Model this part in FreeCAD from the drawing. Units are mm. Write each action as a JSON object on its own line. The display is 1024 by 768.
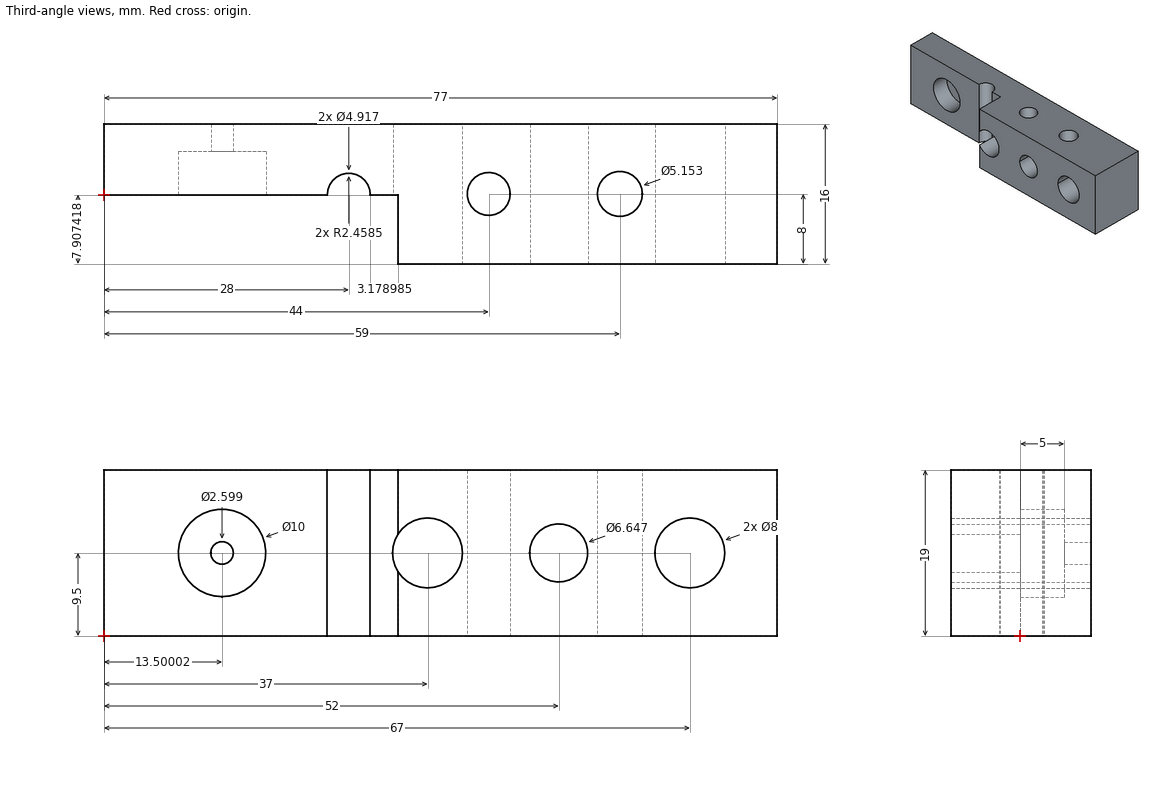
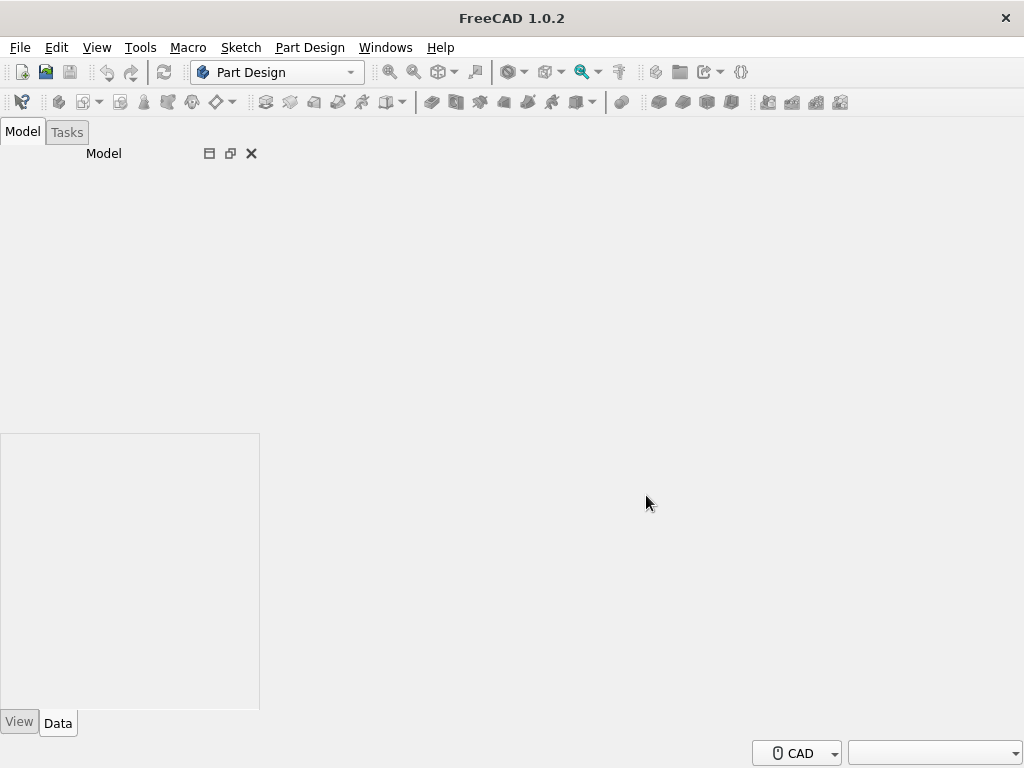
{"action": "left_click", "coordinate": [22, 72]}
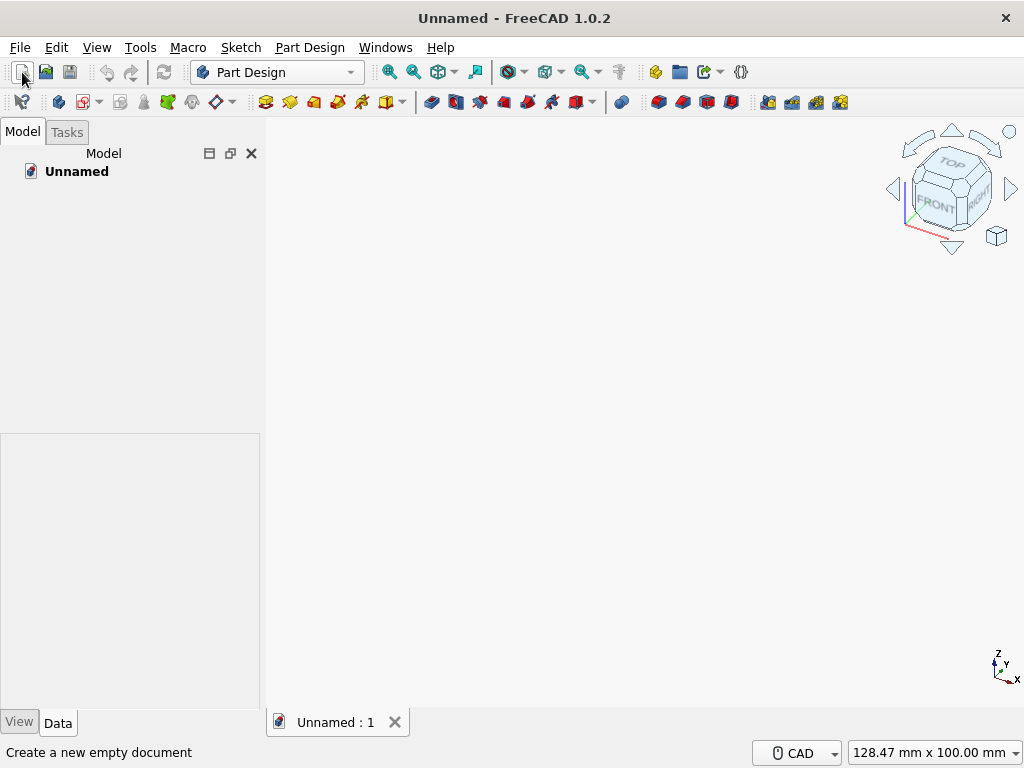
{"action": "left_click", "coordinate": [84, 102]}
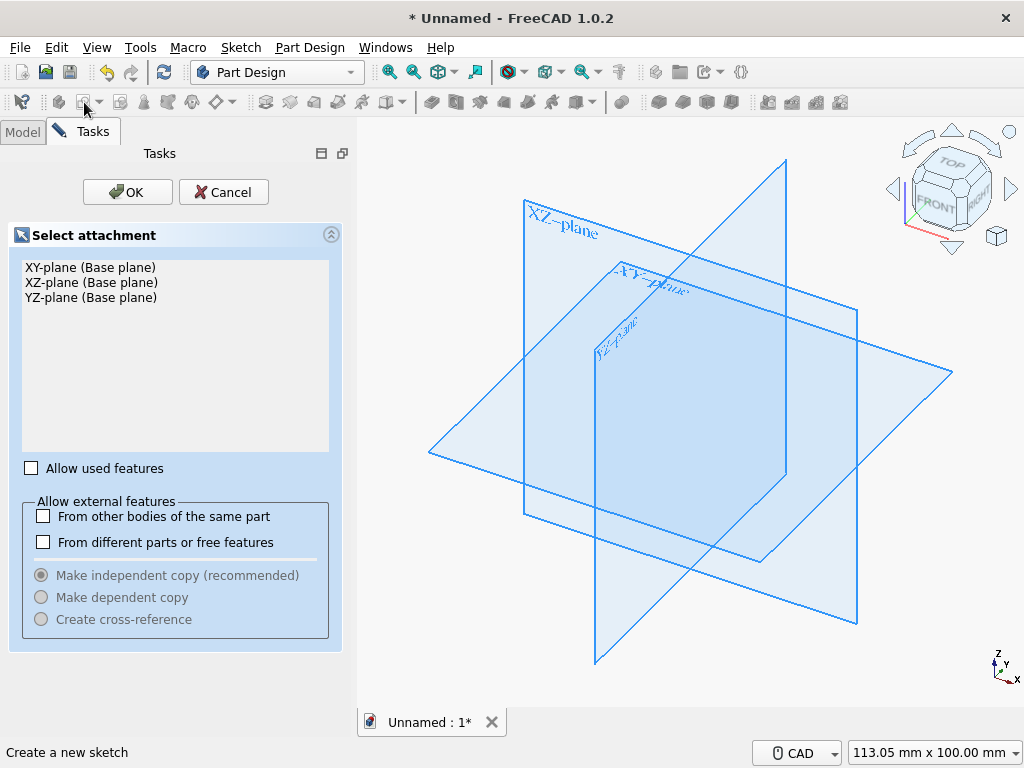
{"action": "left_click", "coordinate": [82, 268]}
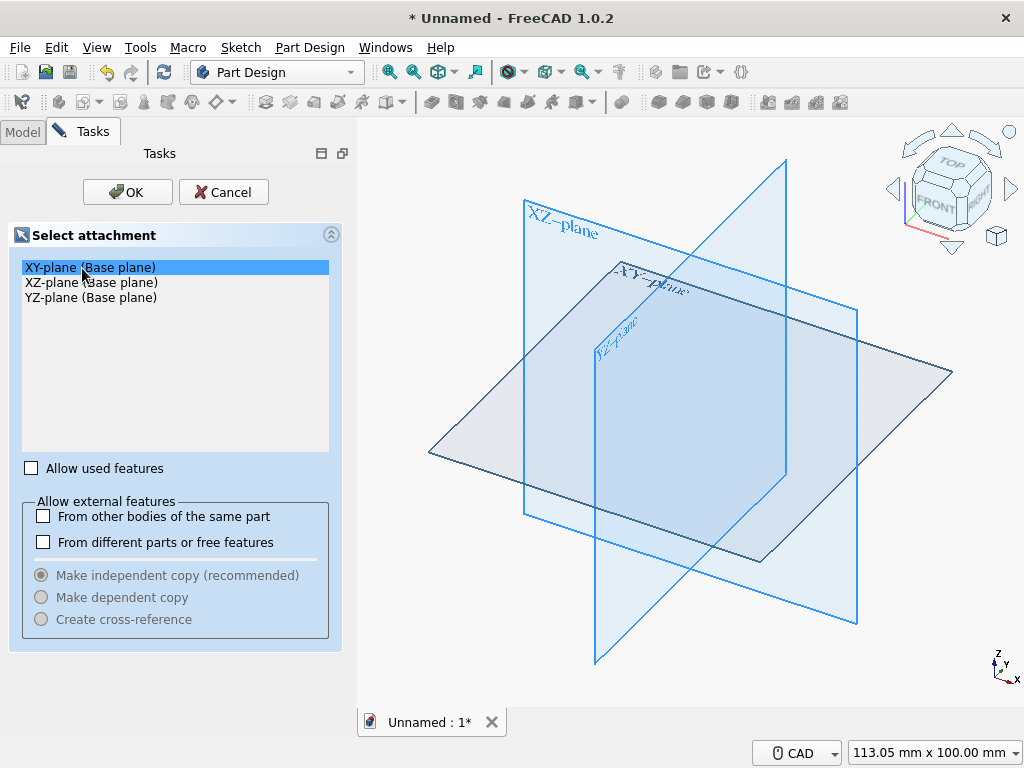
{"action": "left_click", "coordinate": [128, 192]}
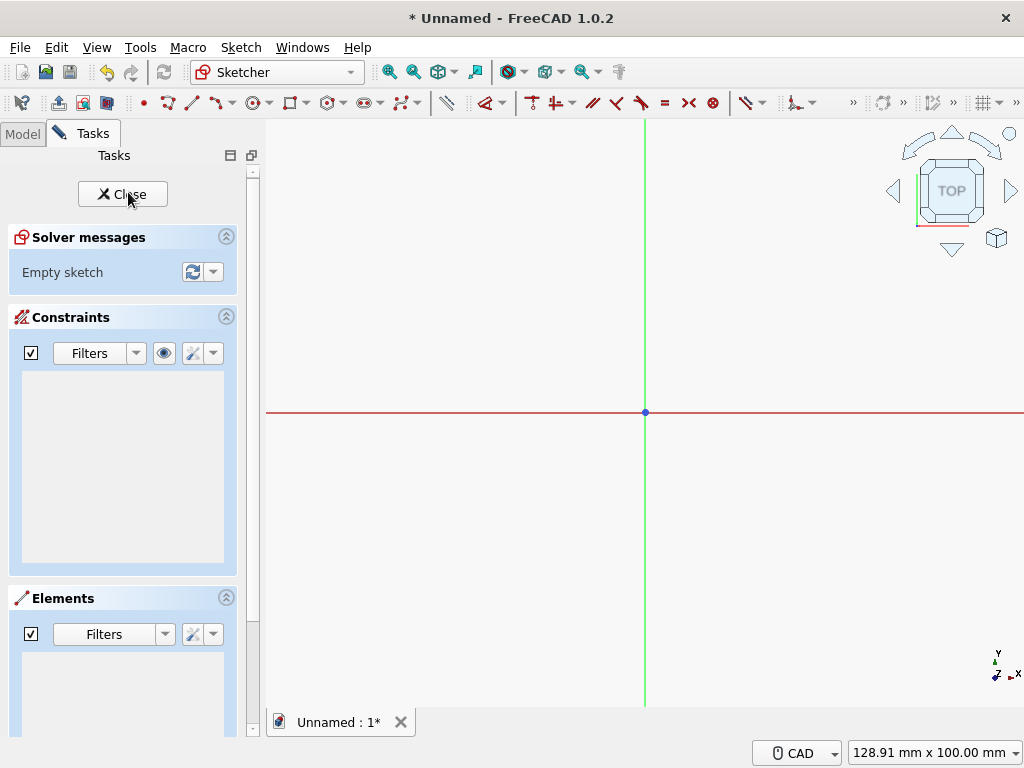
{"action": "scroll", "coordinate": [294, 414], "scroll_direction": "down", "scroll_amount": 2}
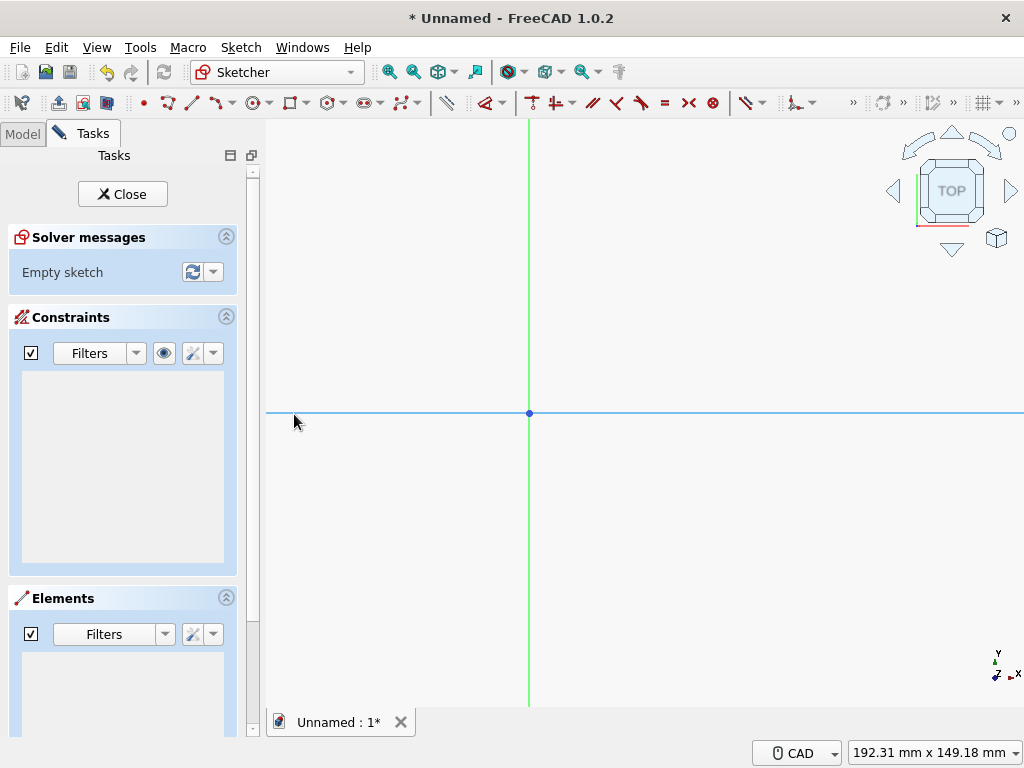
{"action": "key", "text": "g m"}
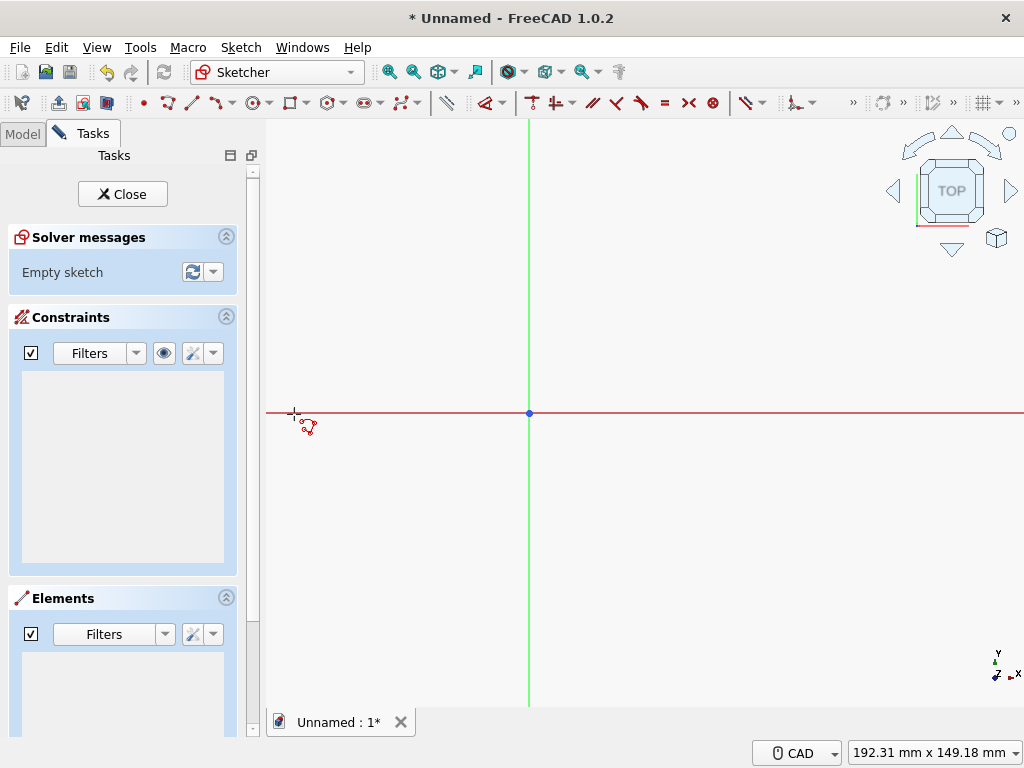
{"action": "left_click", "coordinate": [649, 413]}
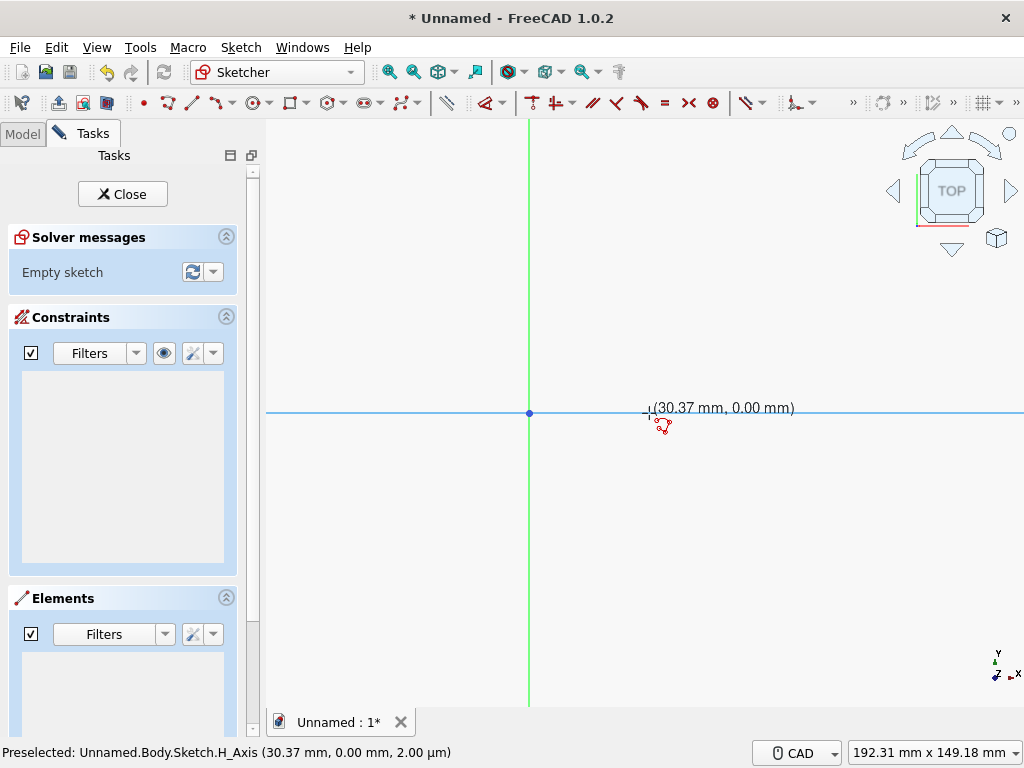
{"action": "scroll", "coordinate": [662, 413], "scroll_direction": "up", "scroll_amount": 2}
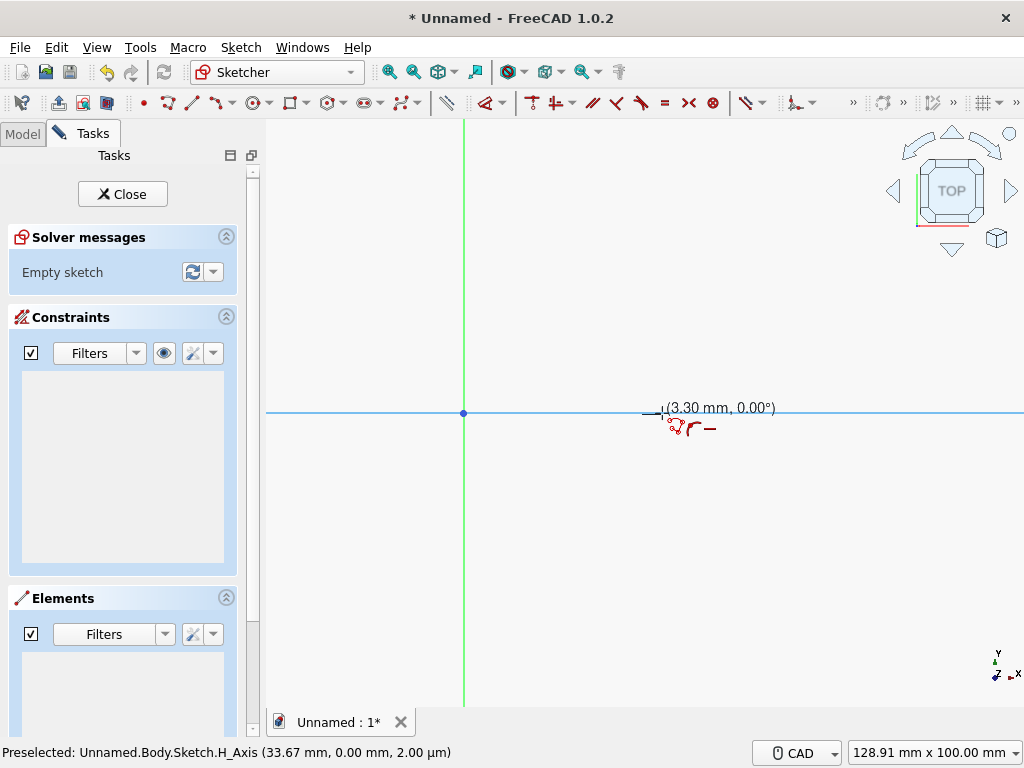
{"action": "left_click", "coordinate": [662, 404]}
{"action": "left_click", "coordinate": [662, 460]}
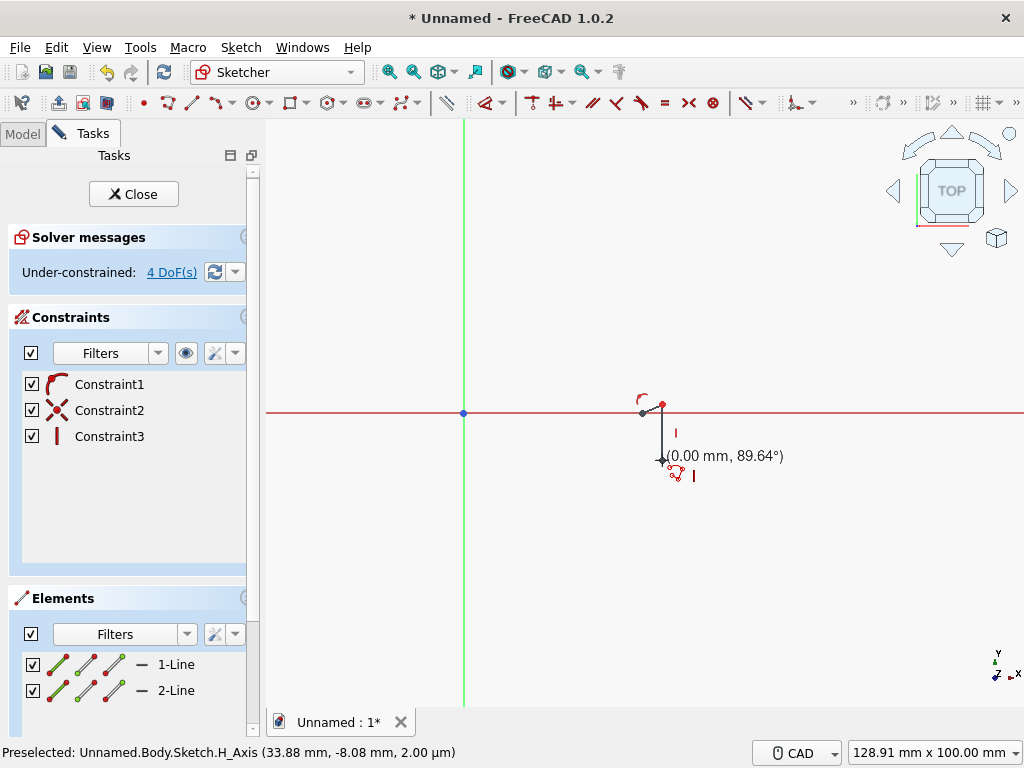
{"action": "scroll", "coordinate": [294, 413], "scroll_direction": "down", "scroll_amount": 1}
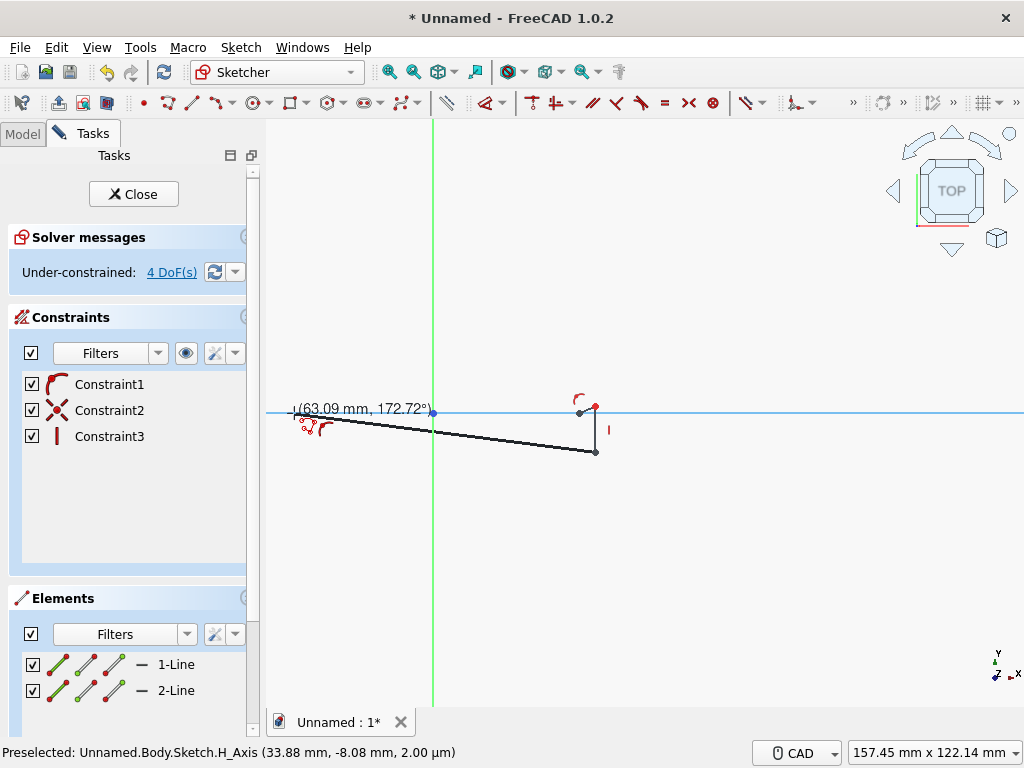
{"action": "left_click", "coordinate": [804, 452]}
{"action": "left_click", "coordinate": [804, 375]}
{"action": "left_click", "coordinate": [433, 375]}
{"action": "left_click", "coordinate": [433, 413]}
{"action": "left_click", "coordinate": [556, 404]}
{"action": "right_click", "coordinate": [556, 404]}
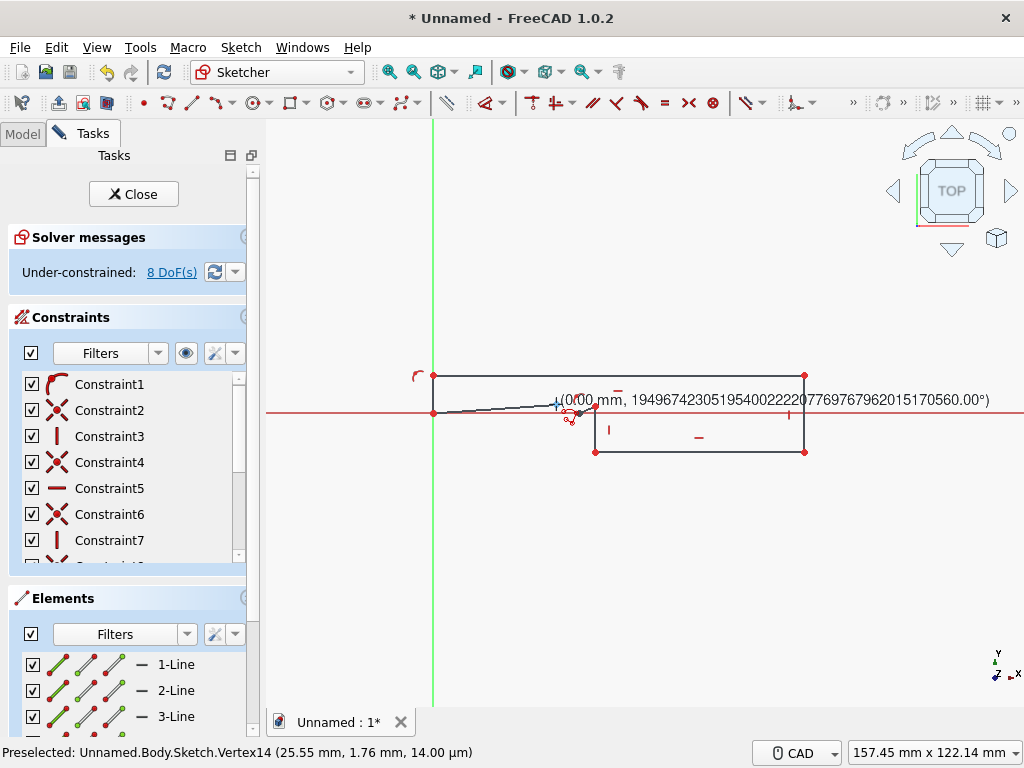
{"action": "key", "text": "g 3 a"}